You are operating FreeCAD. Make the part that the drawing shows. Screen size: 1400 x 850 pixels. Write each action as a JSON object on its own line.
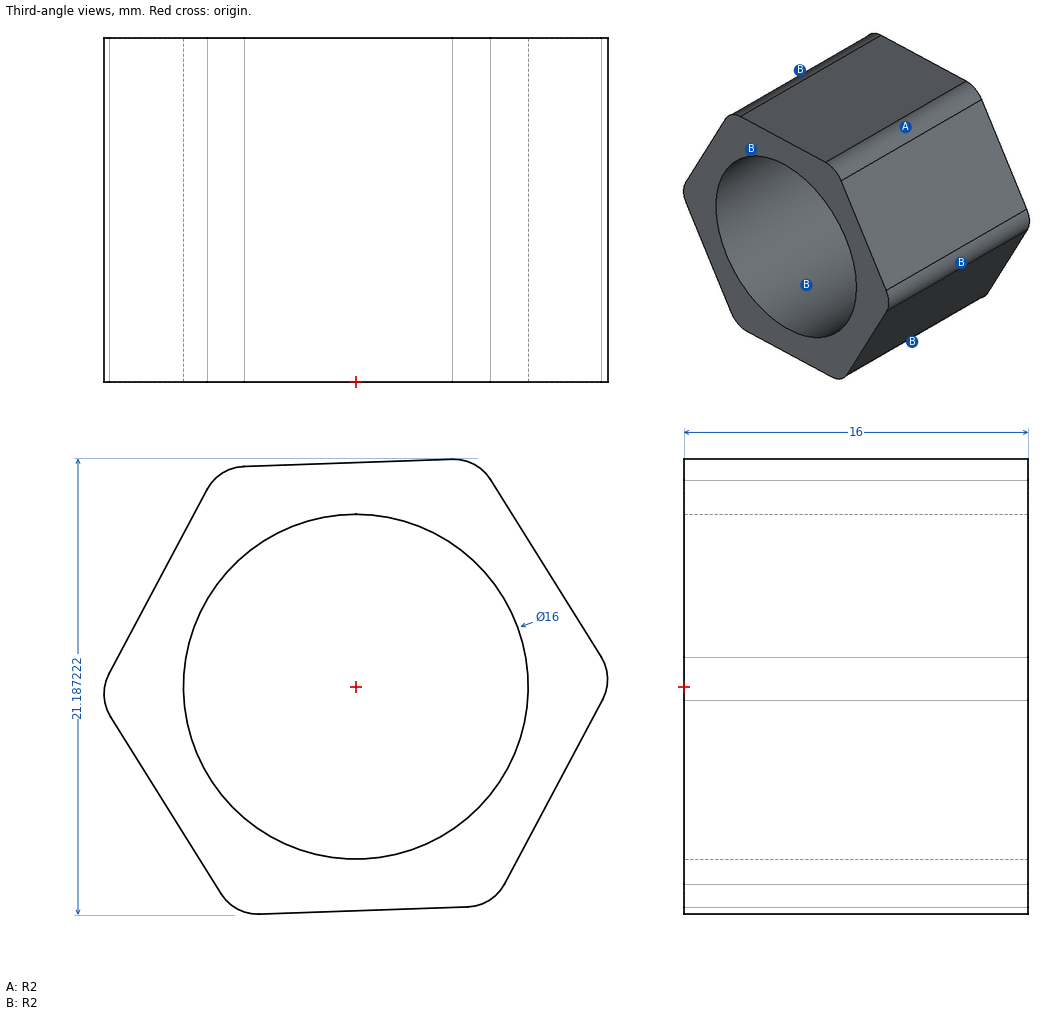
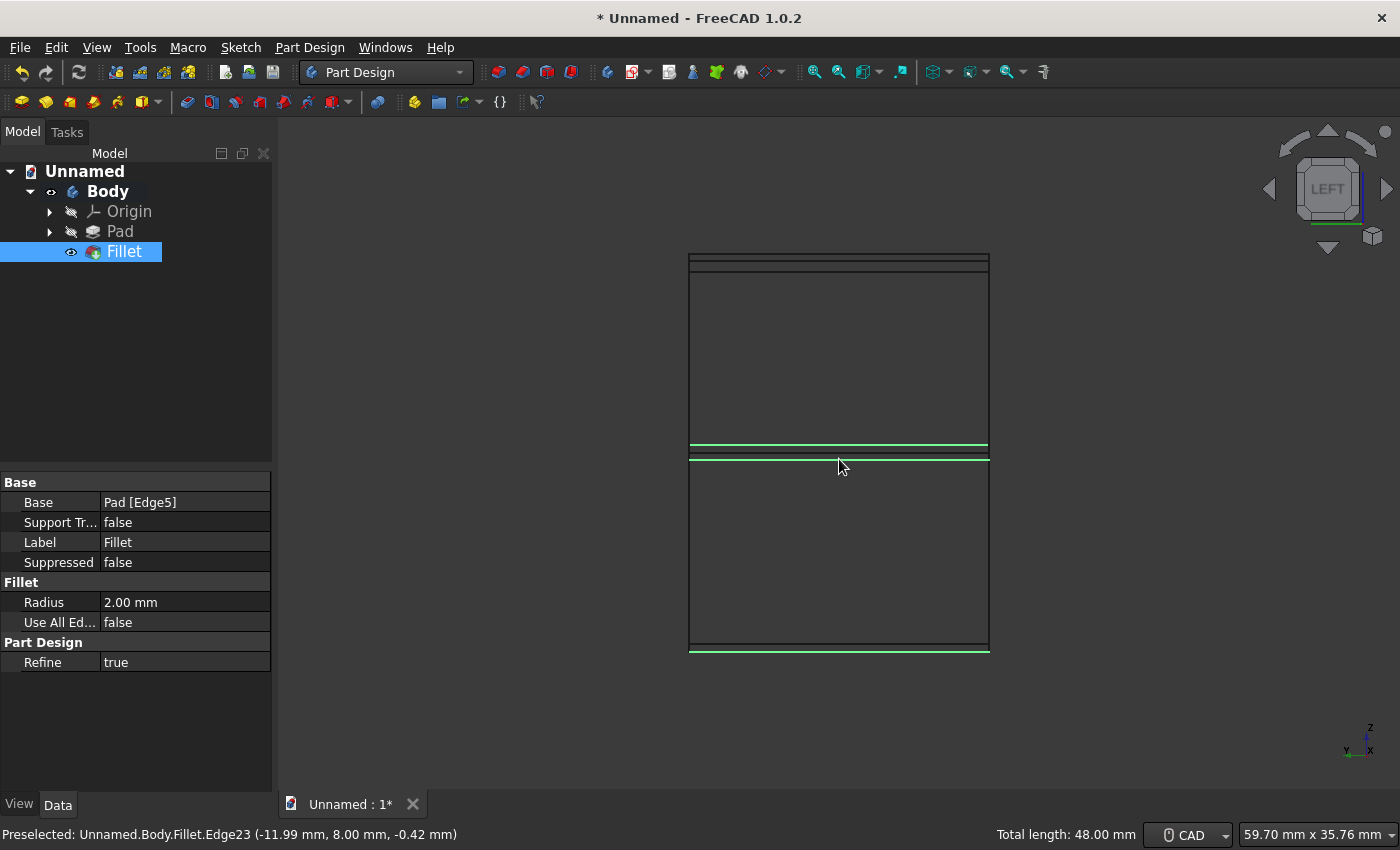
{"action": "key", "text": "0"}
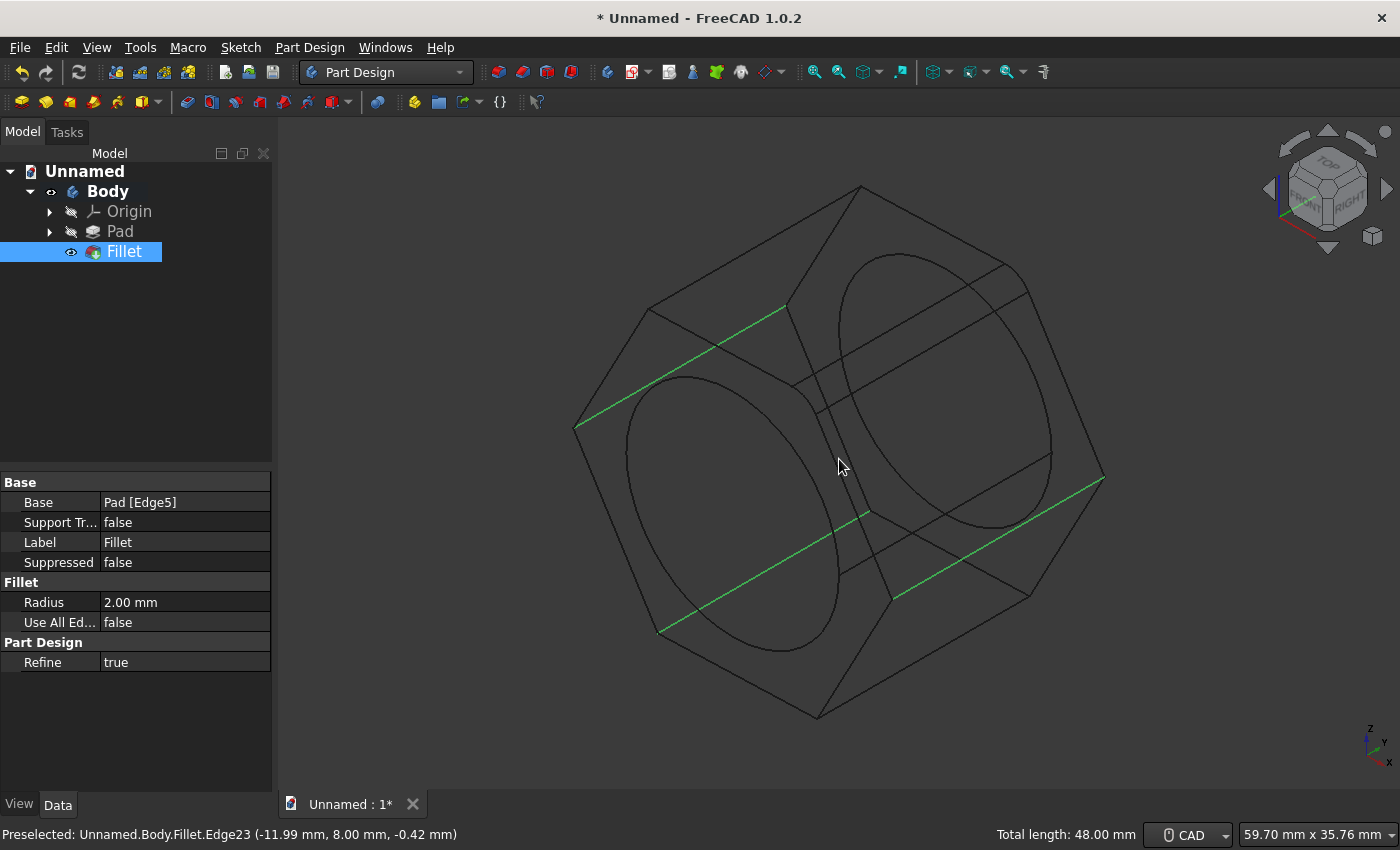
{"action": "left_click", "coordinate": [755, 247], "text": "ctrl"}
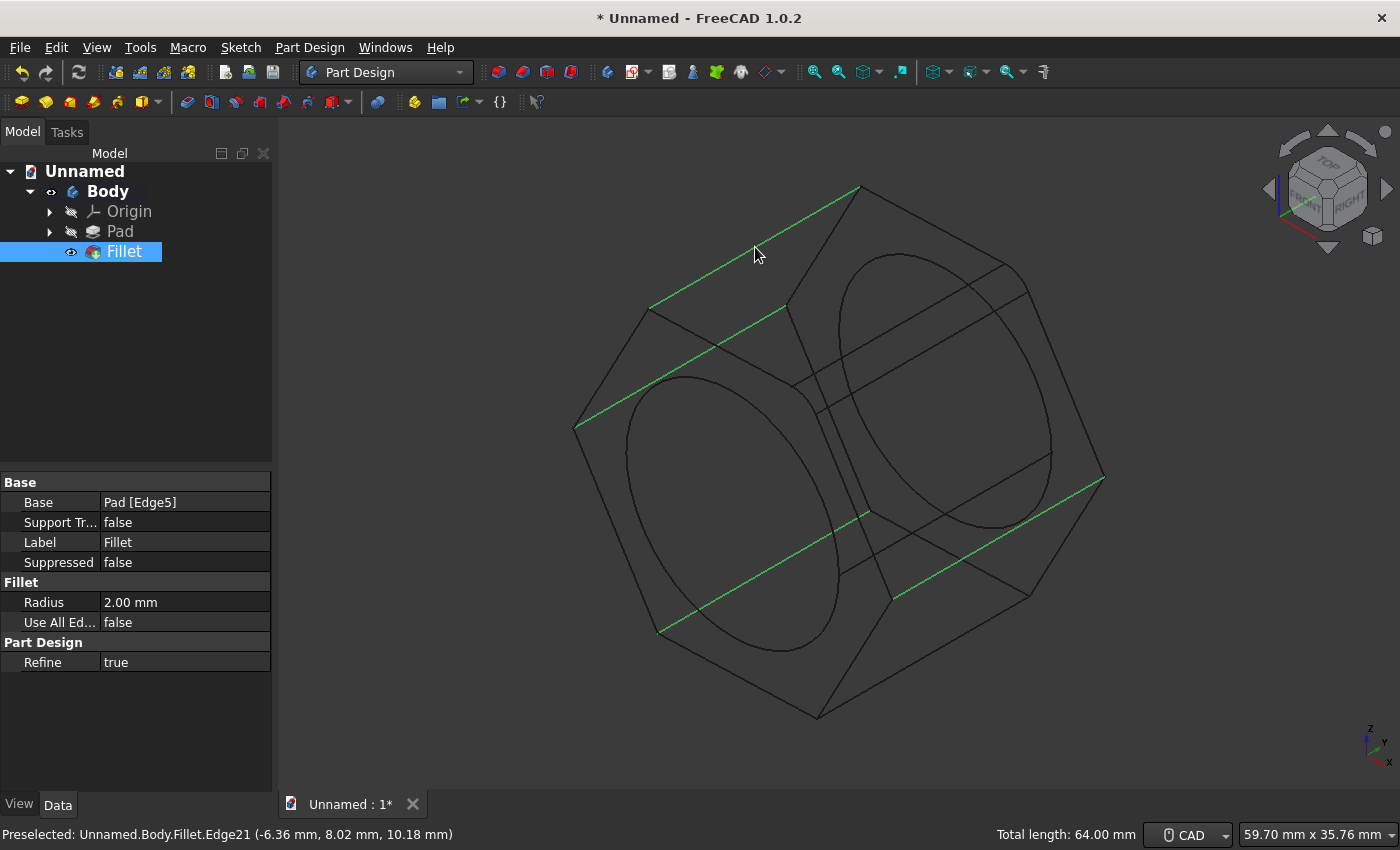
{"action": "left_click", "coordinate": [923, 657], "text": "ctrl"}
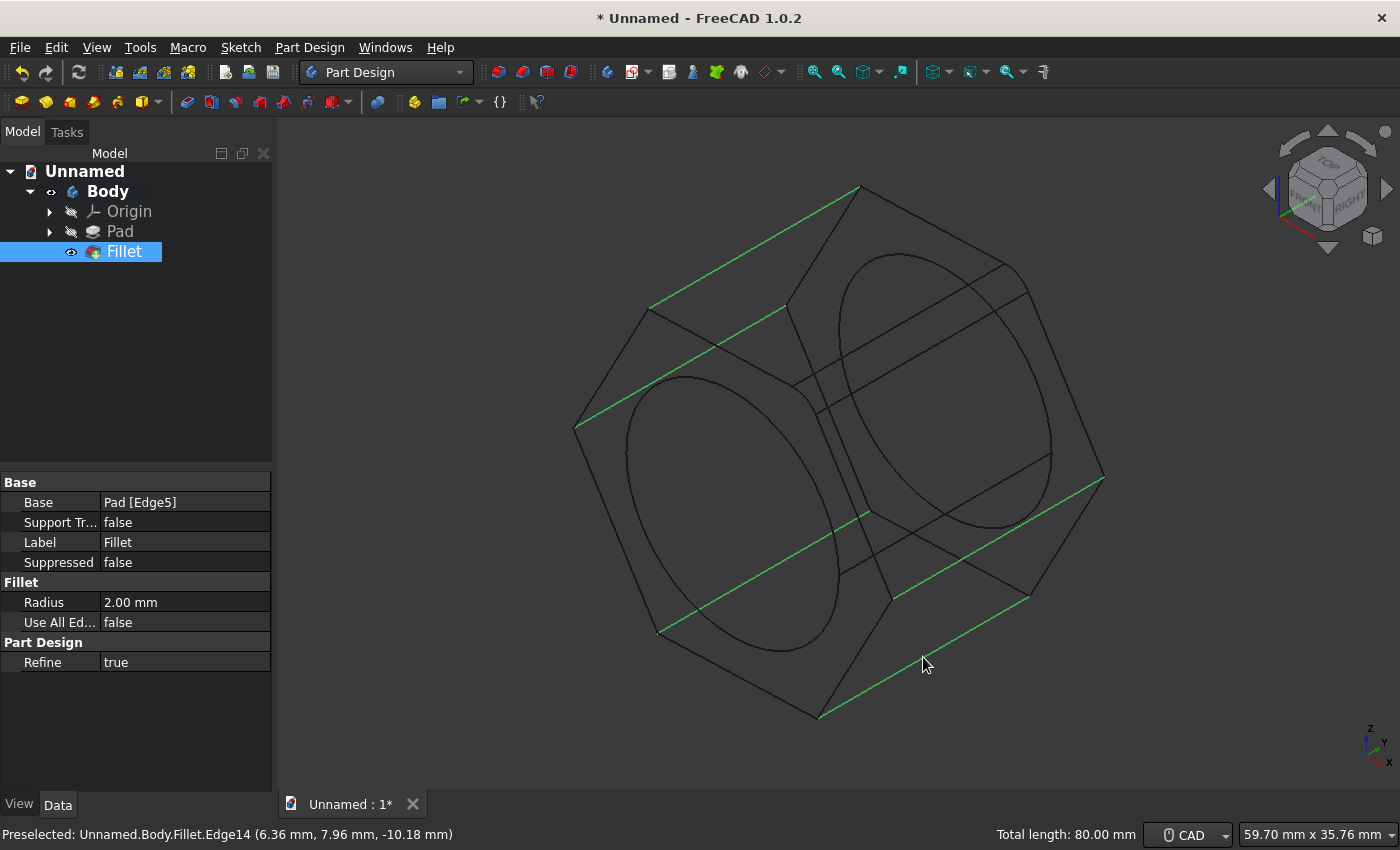
{"action": "key", "text": "v 1"}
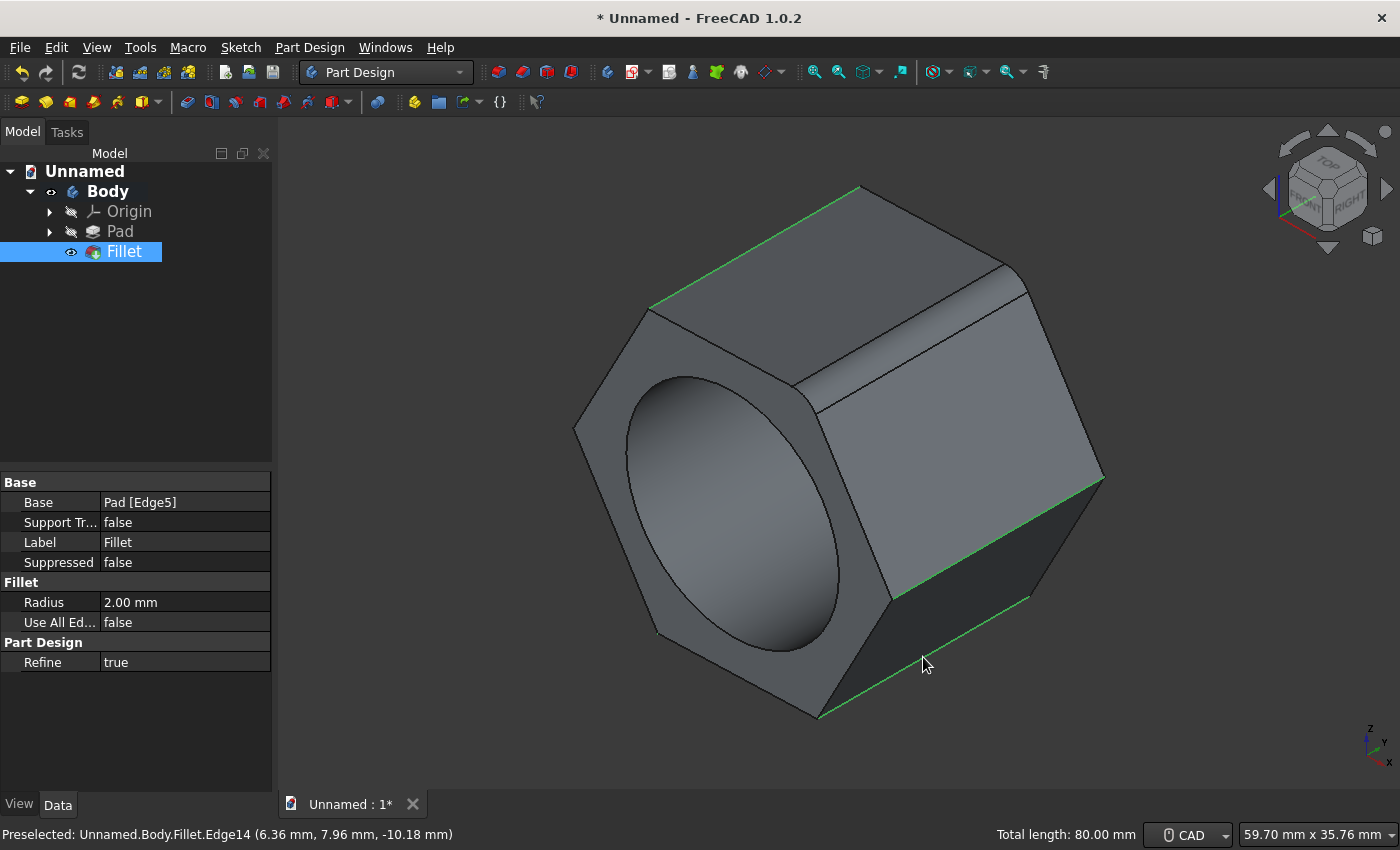
{"action": "left_click", "coordinate": [500, 72]}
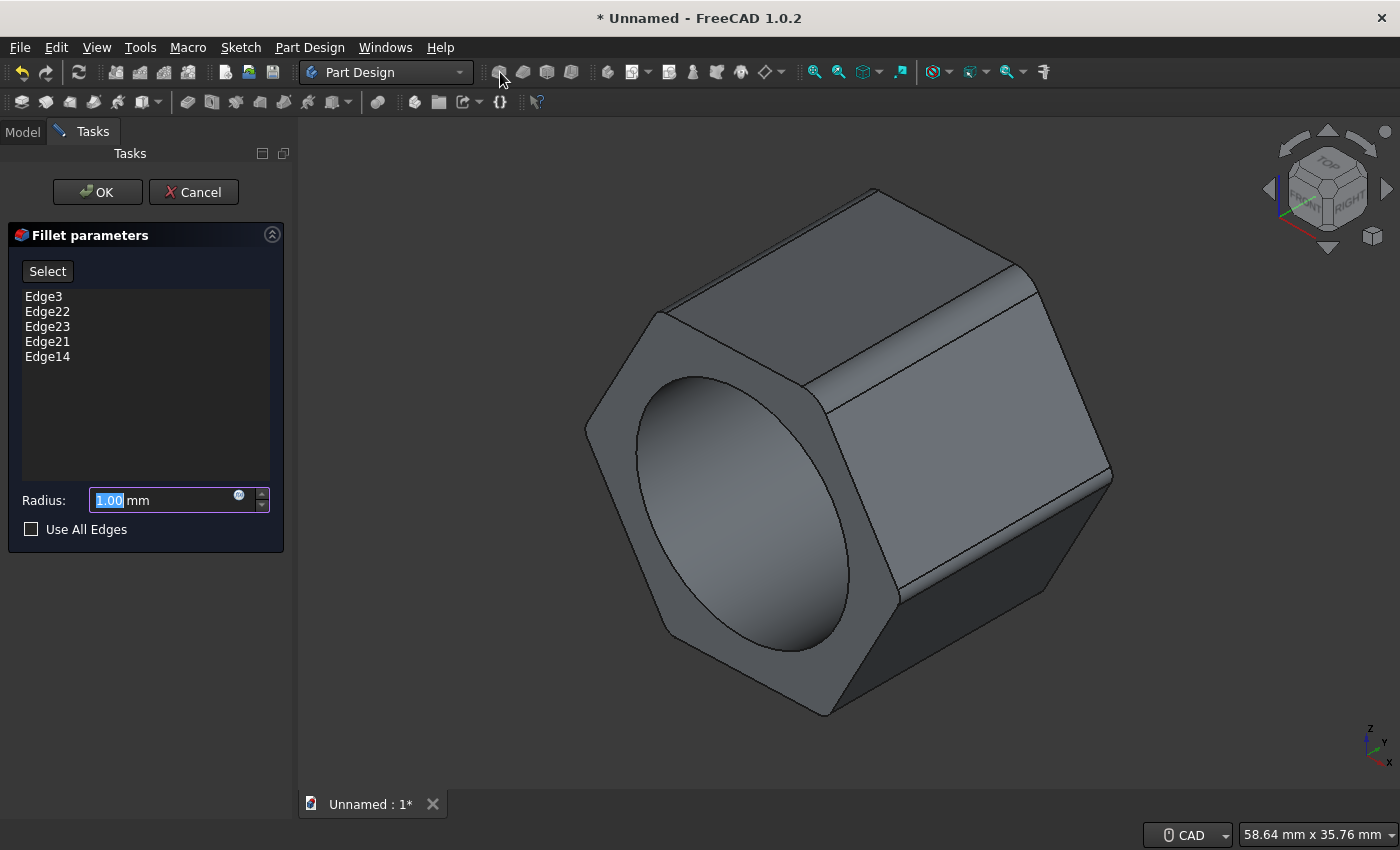
{"action": "type", "text": "2"}
{"action": "key", "text": "Tab"}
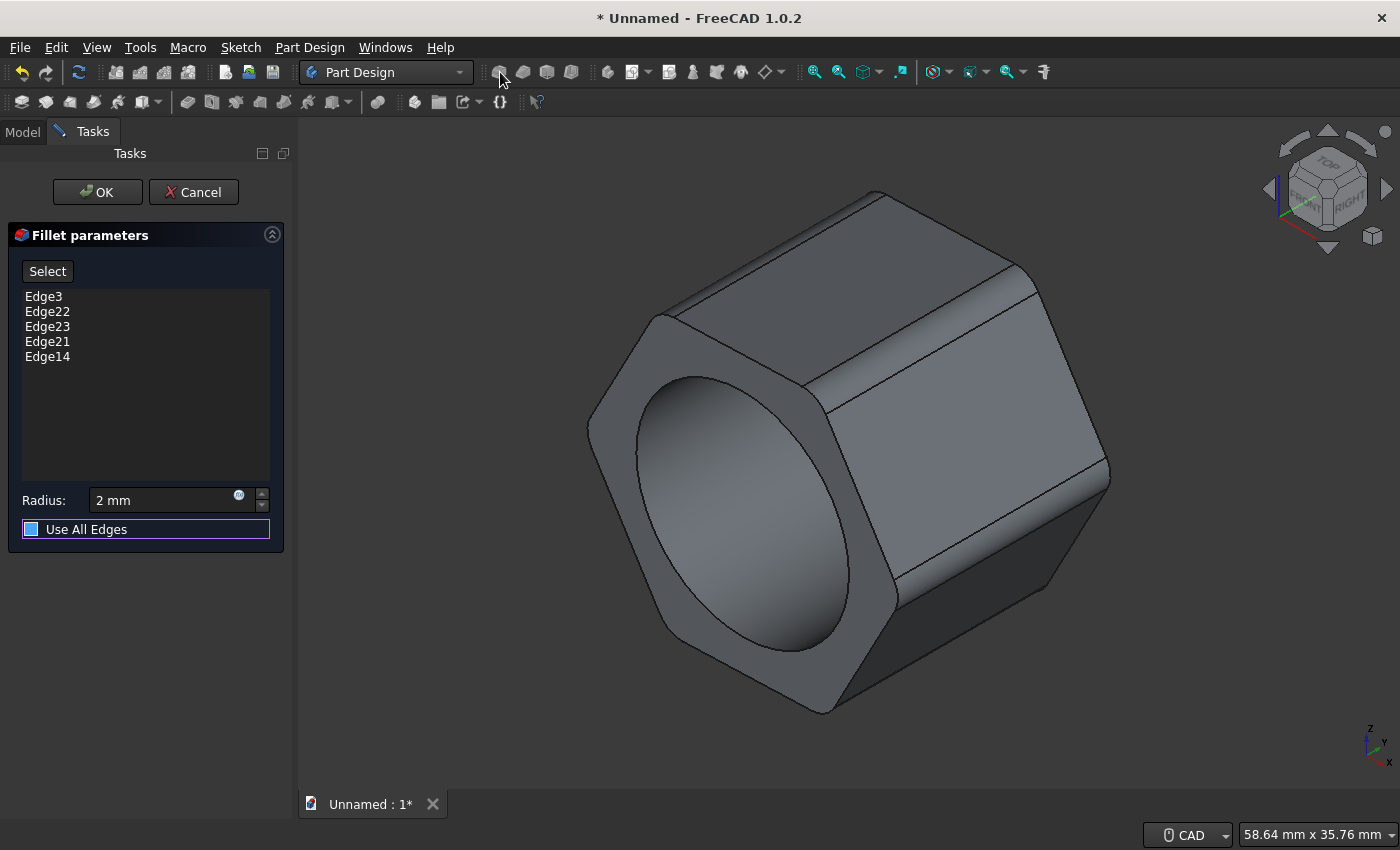
{"action": "left_click", "coordinate": [98, 192]}